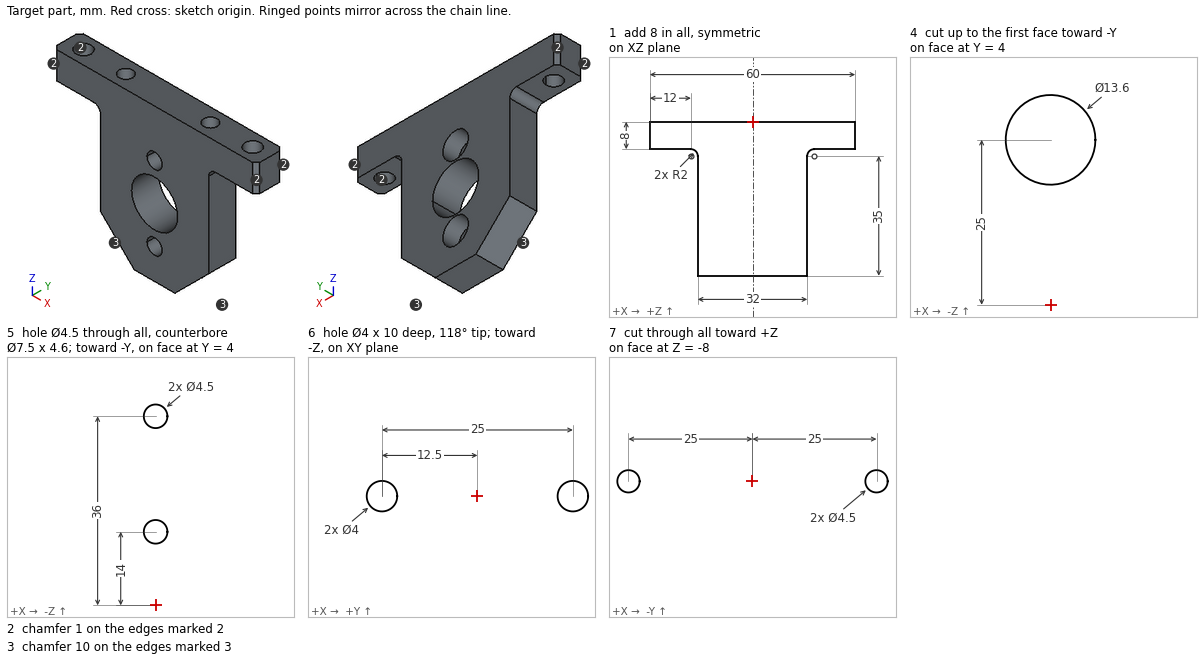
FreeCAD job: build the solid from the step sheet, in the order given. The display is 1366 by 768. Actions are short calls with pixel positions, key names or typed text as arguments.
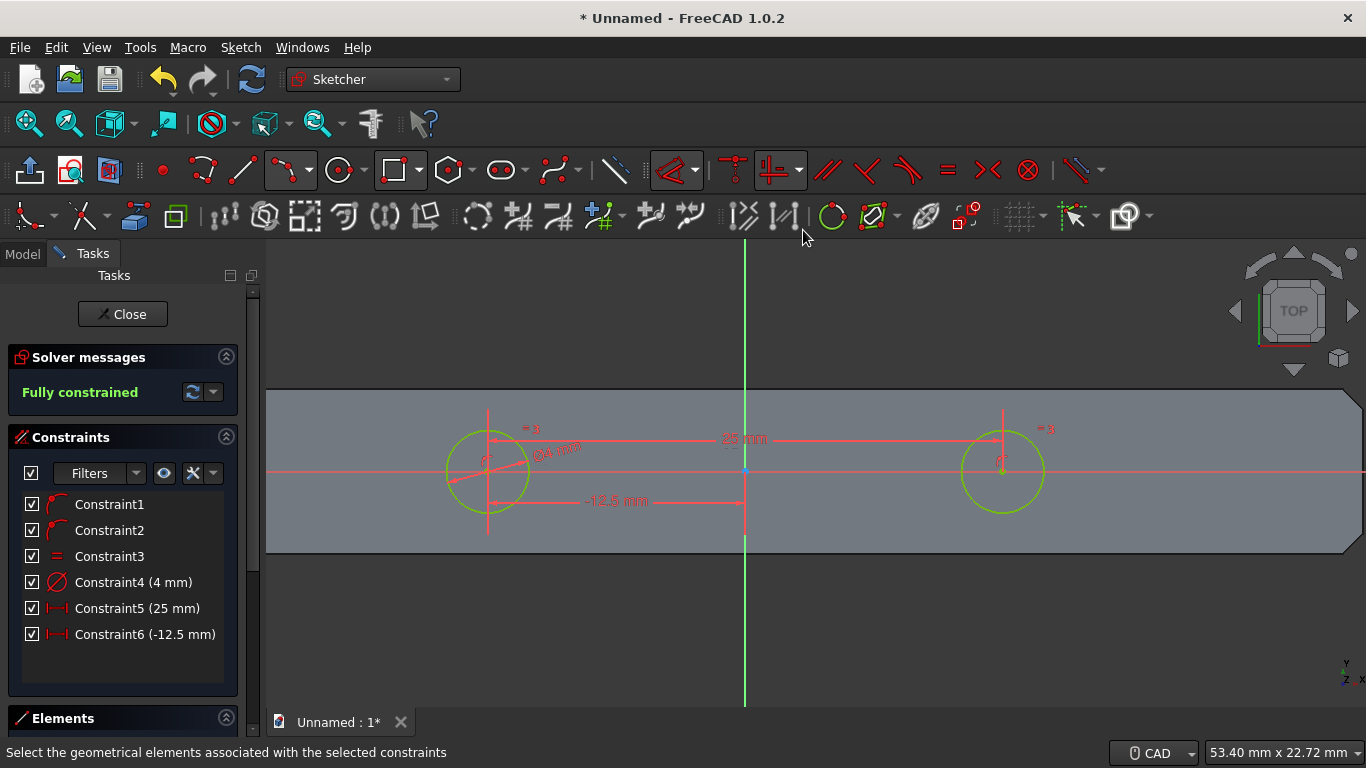
click(123, 314)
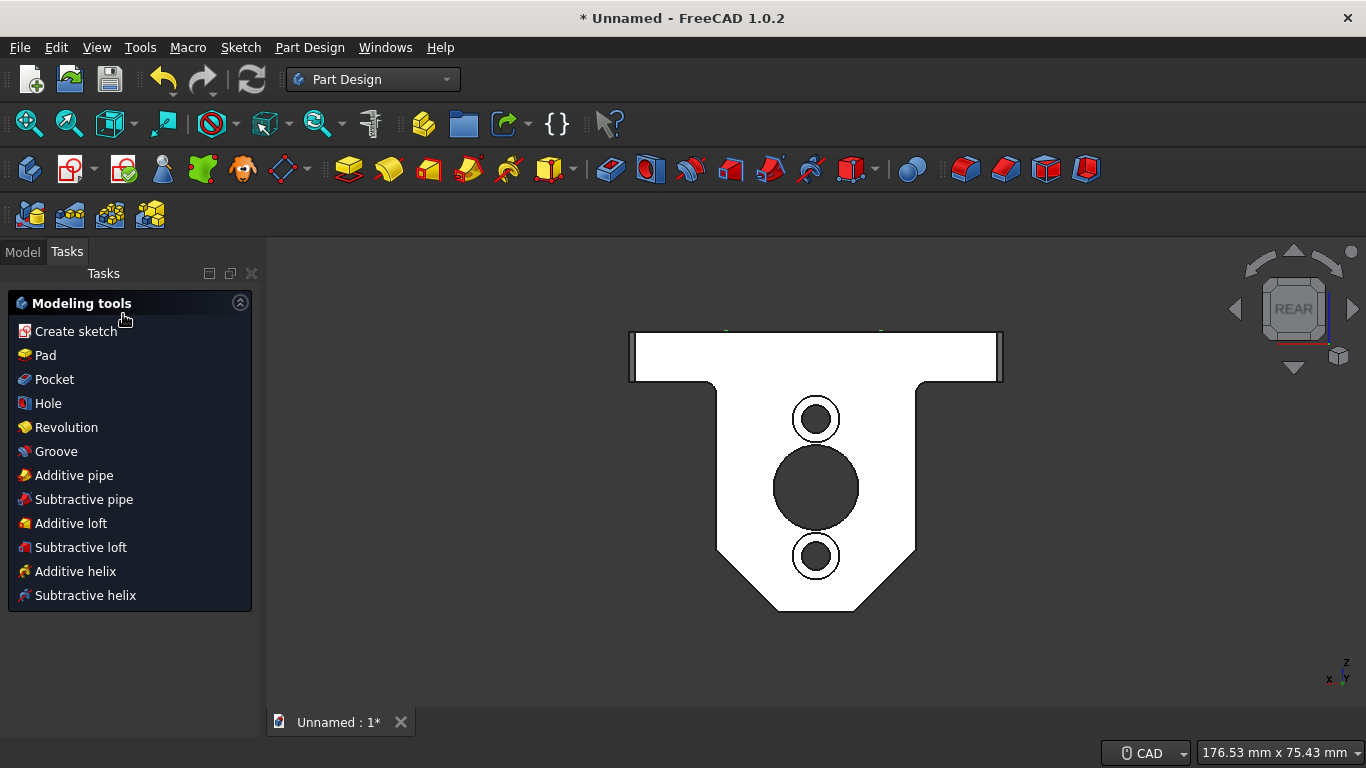
click(652, 170)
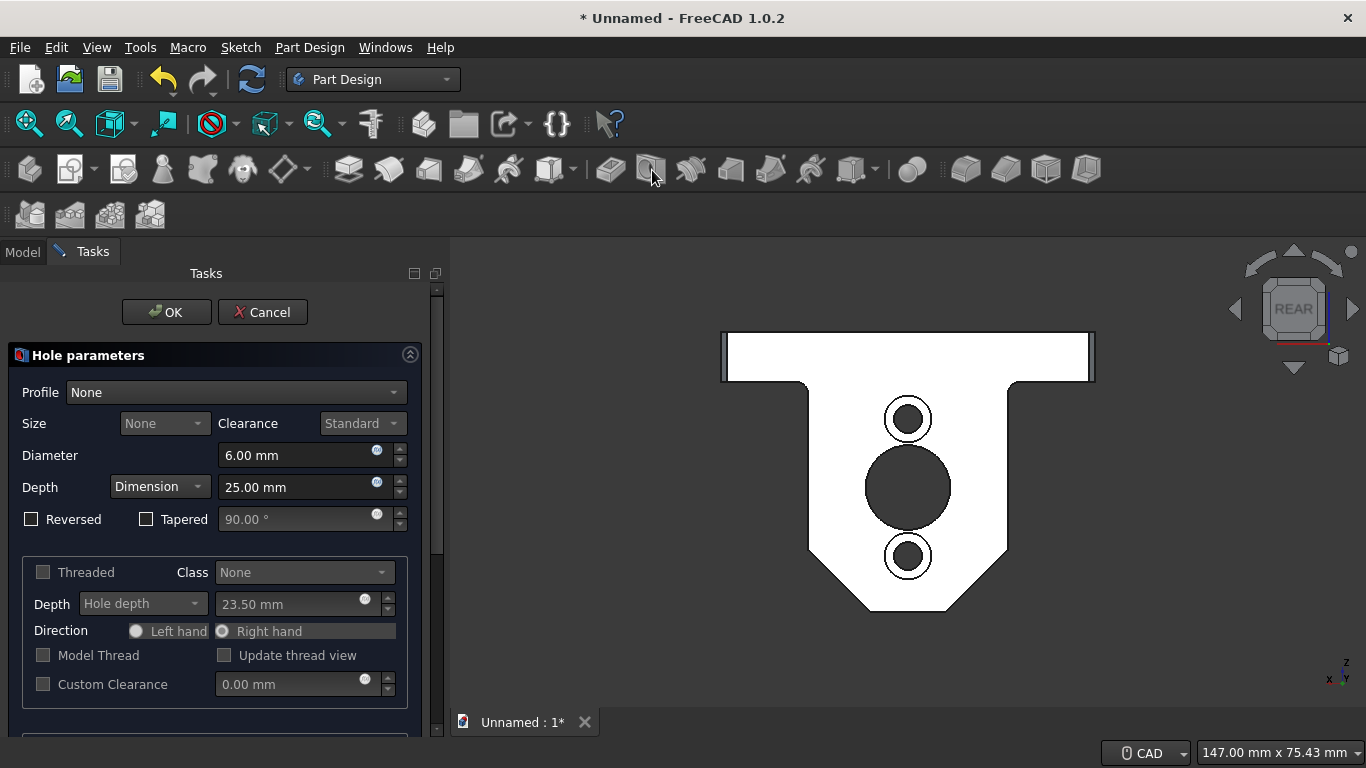
triple_click(305, 455)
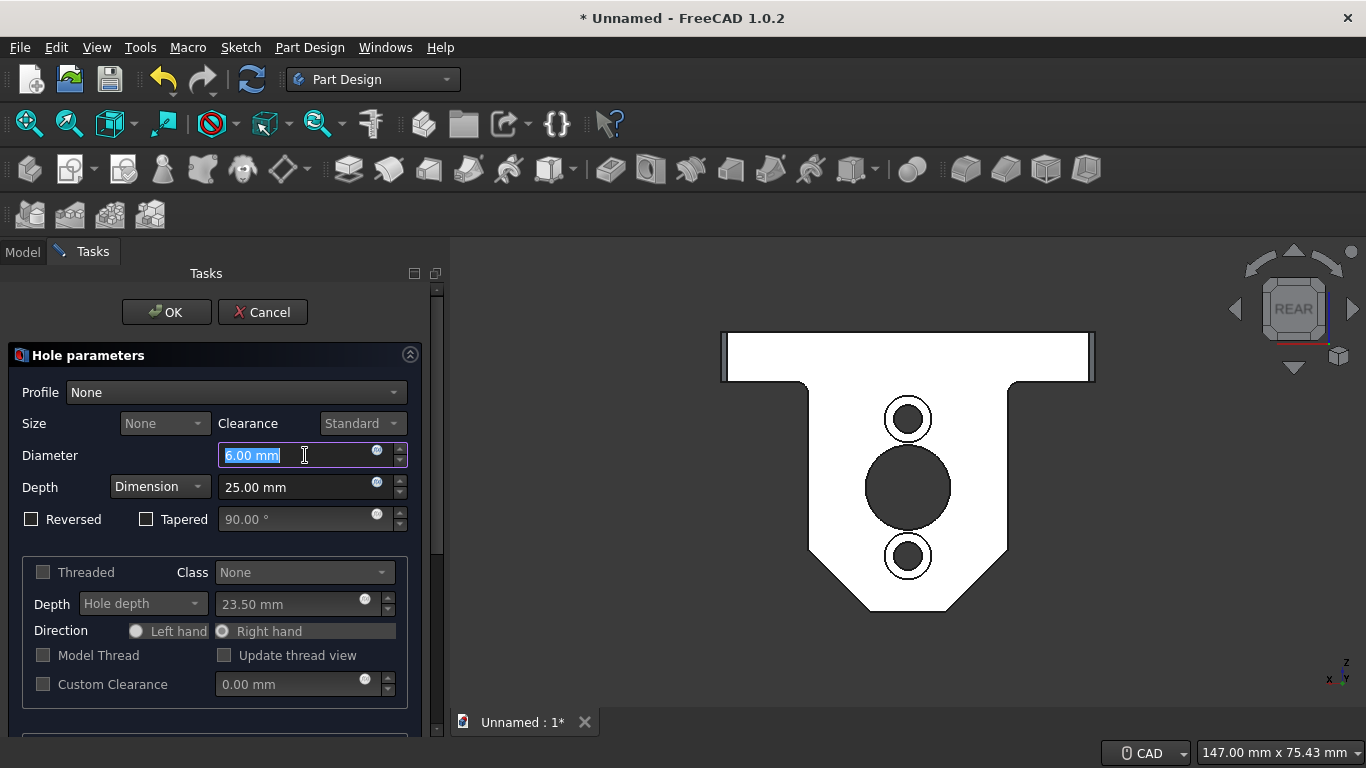
text(4)
key(Tab)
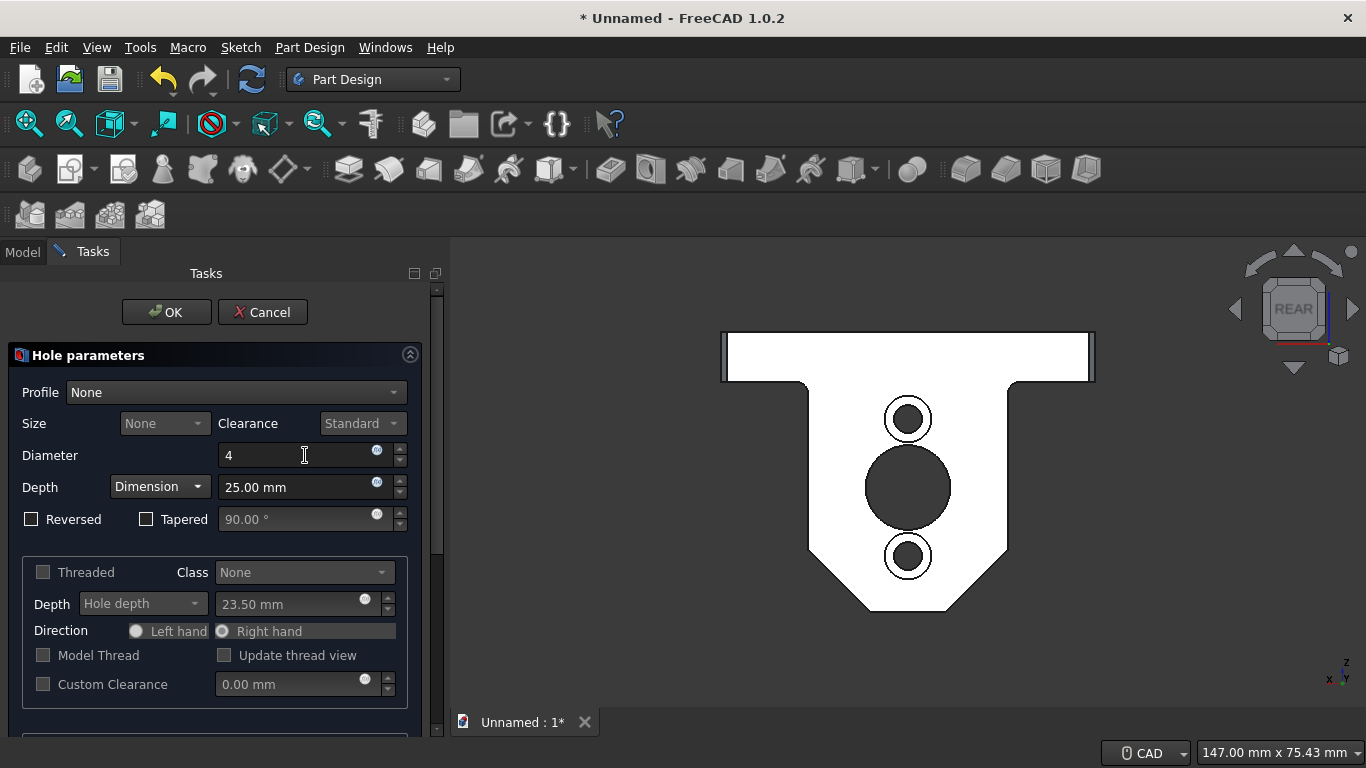
triple_click(305, 487)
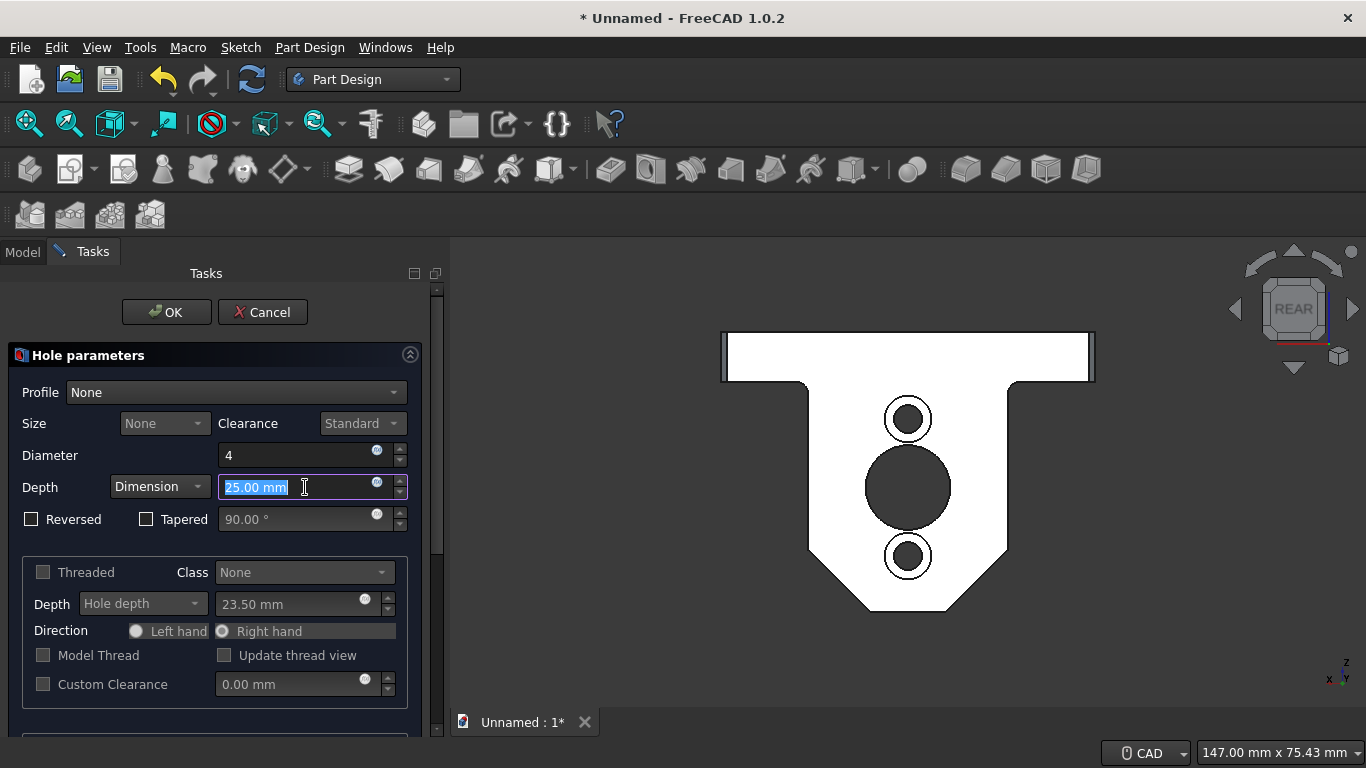
text(10)
key(Tab)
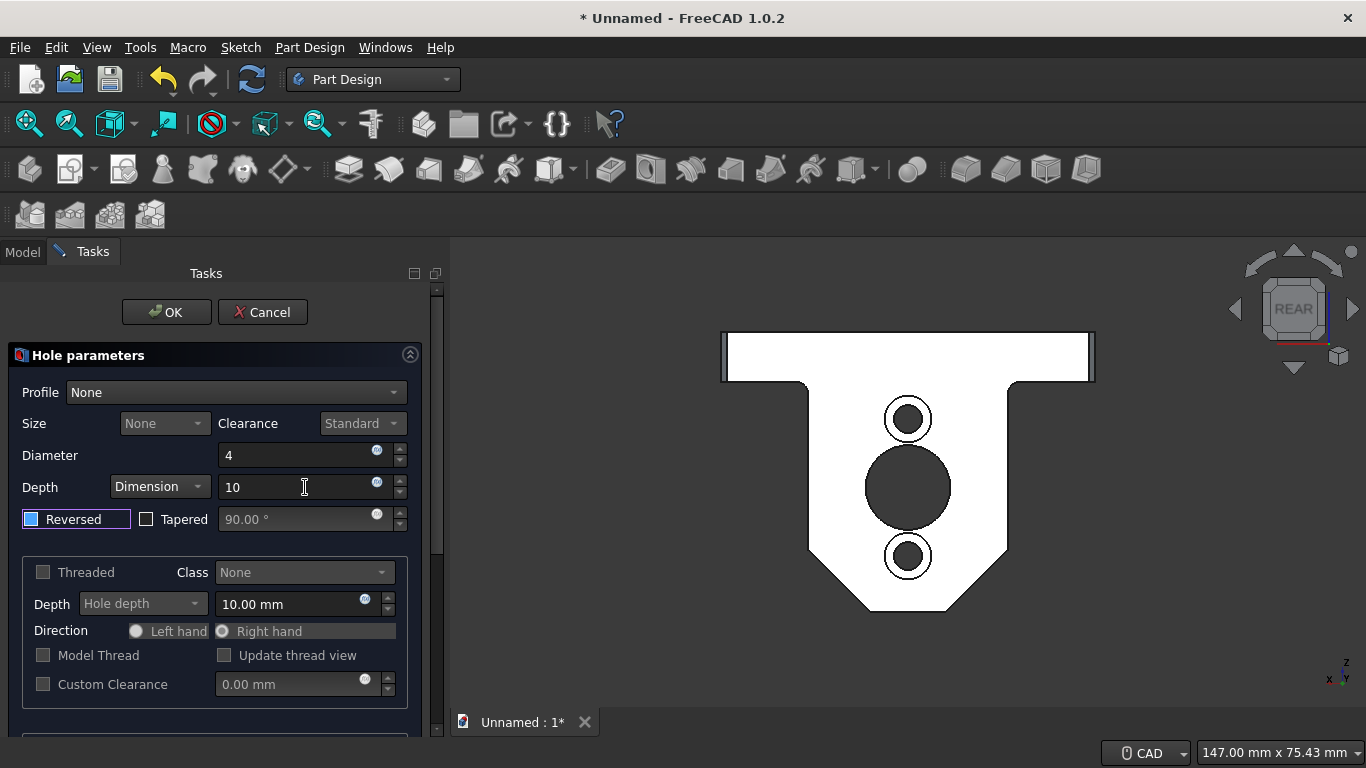
click(167, 312)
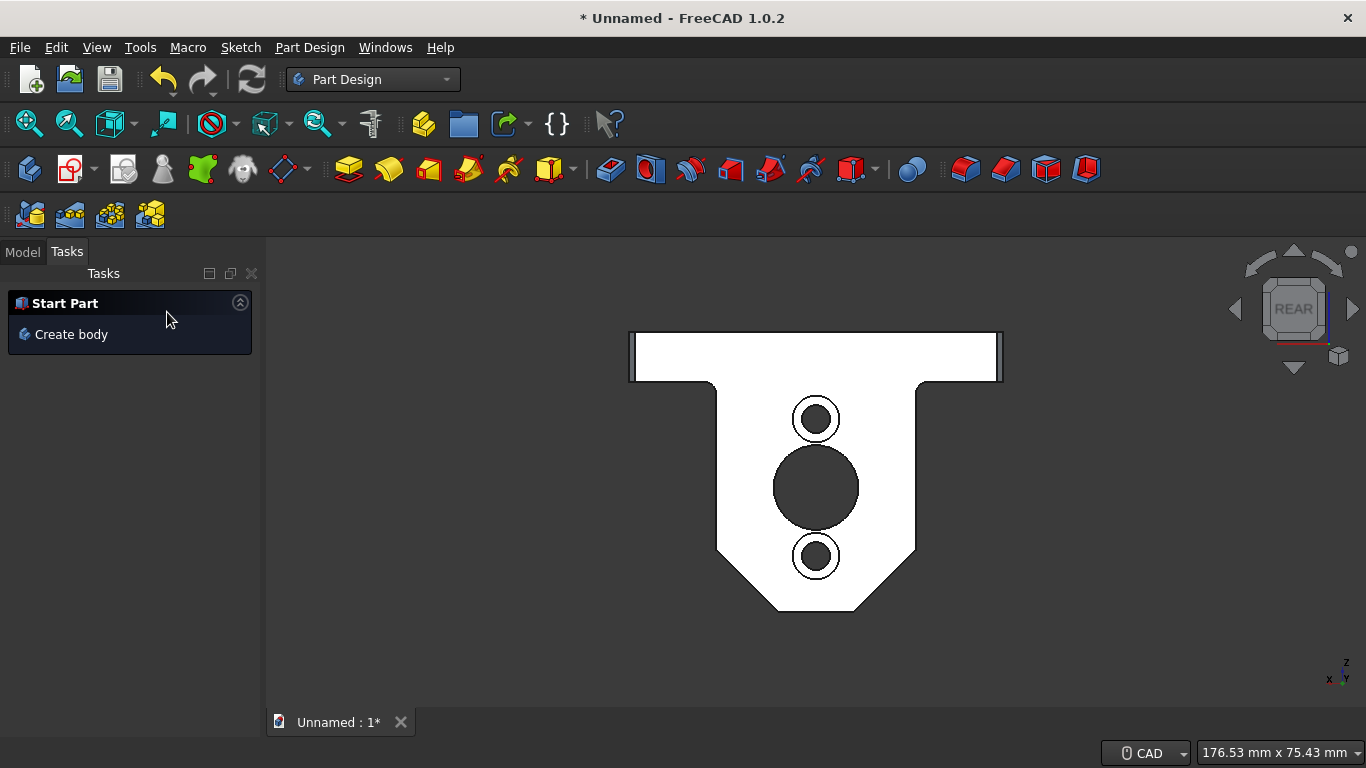
key(5)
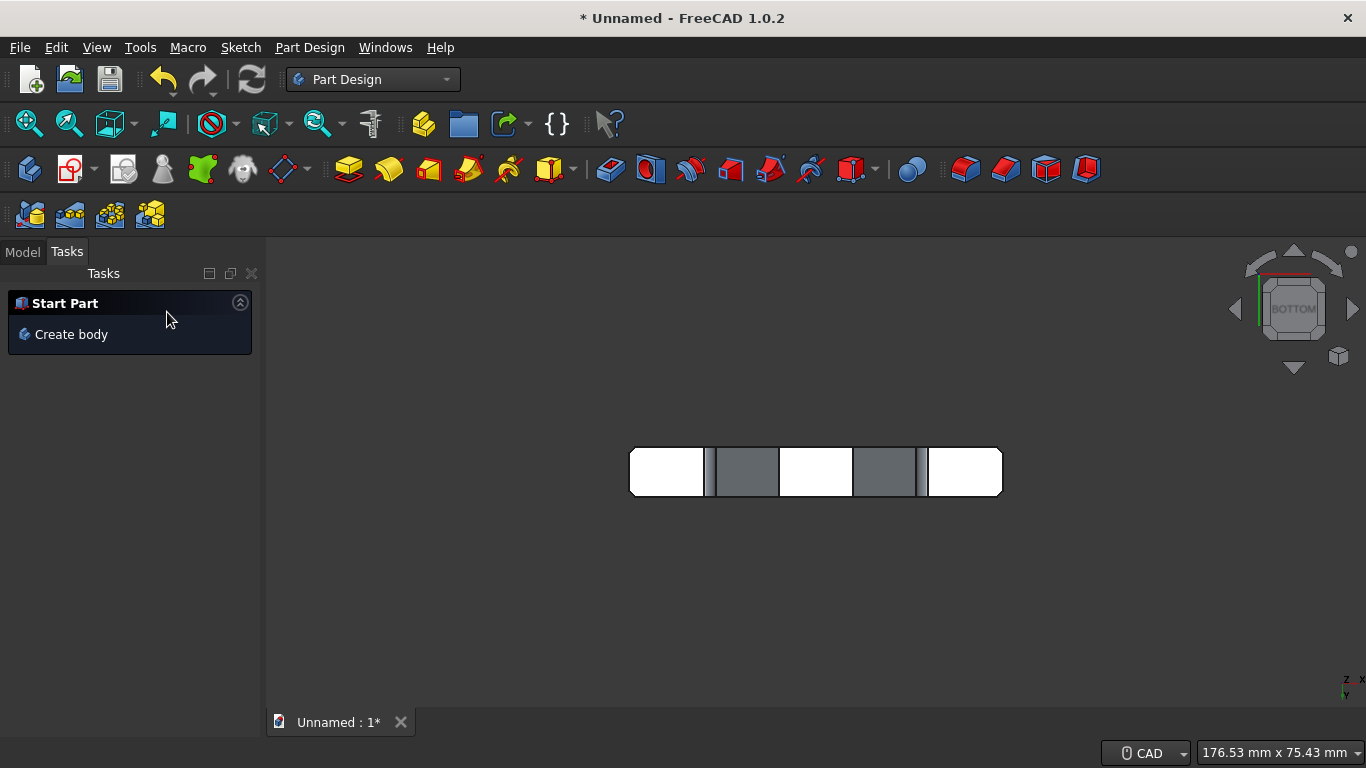
click(30, 124)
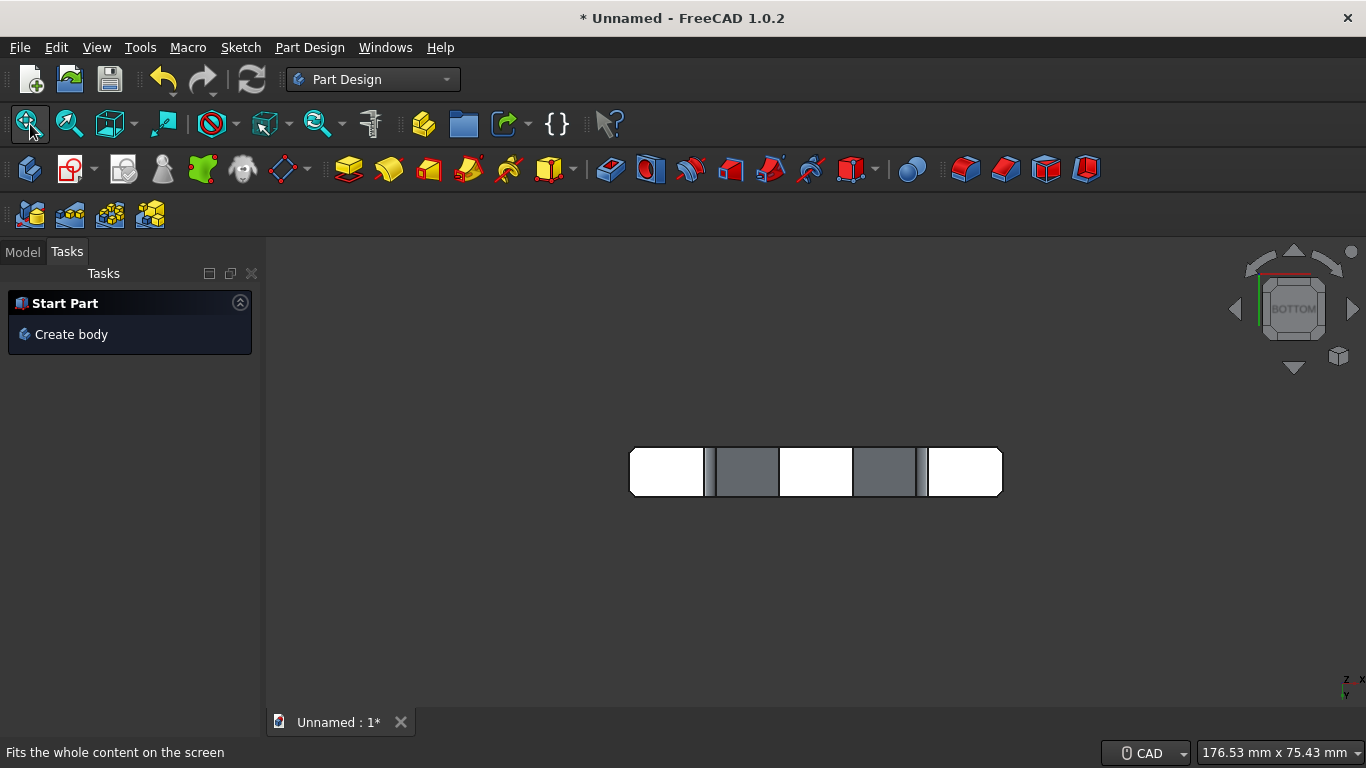
click(677, 471)